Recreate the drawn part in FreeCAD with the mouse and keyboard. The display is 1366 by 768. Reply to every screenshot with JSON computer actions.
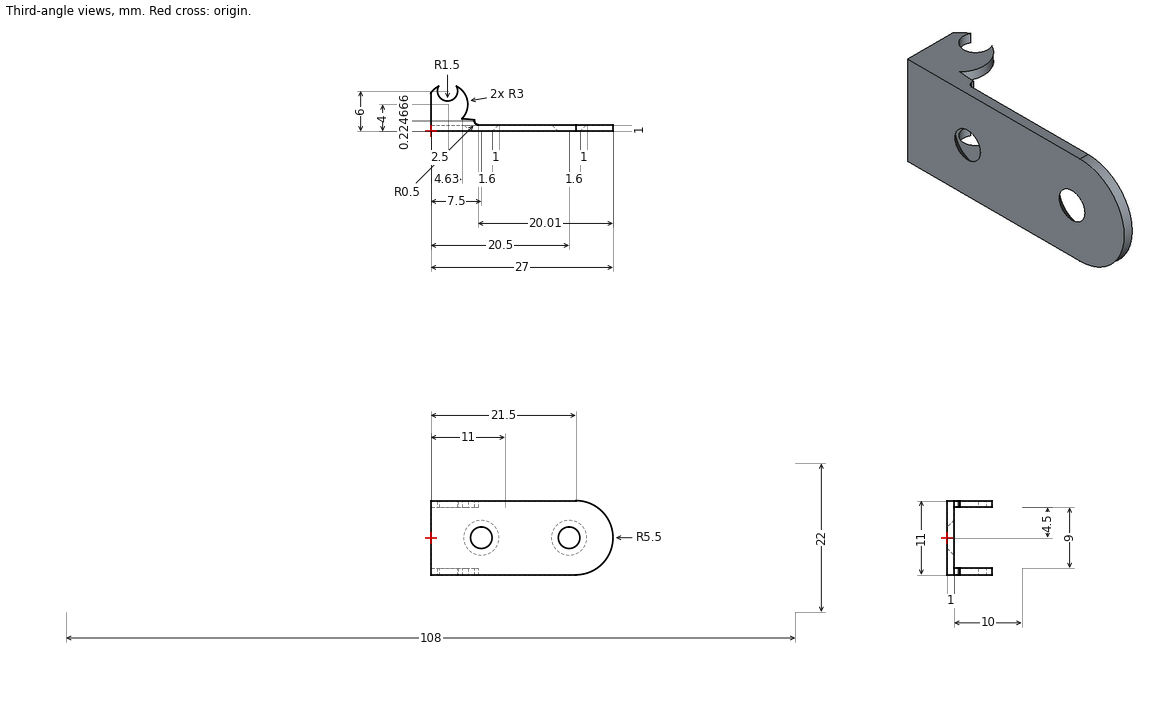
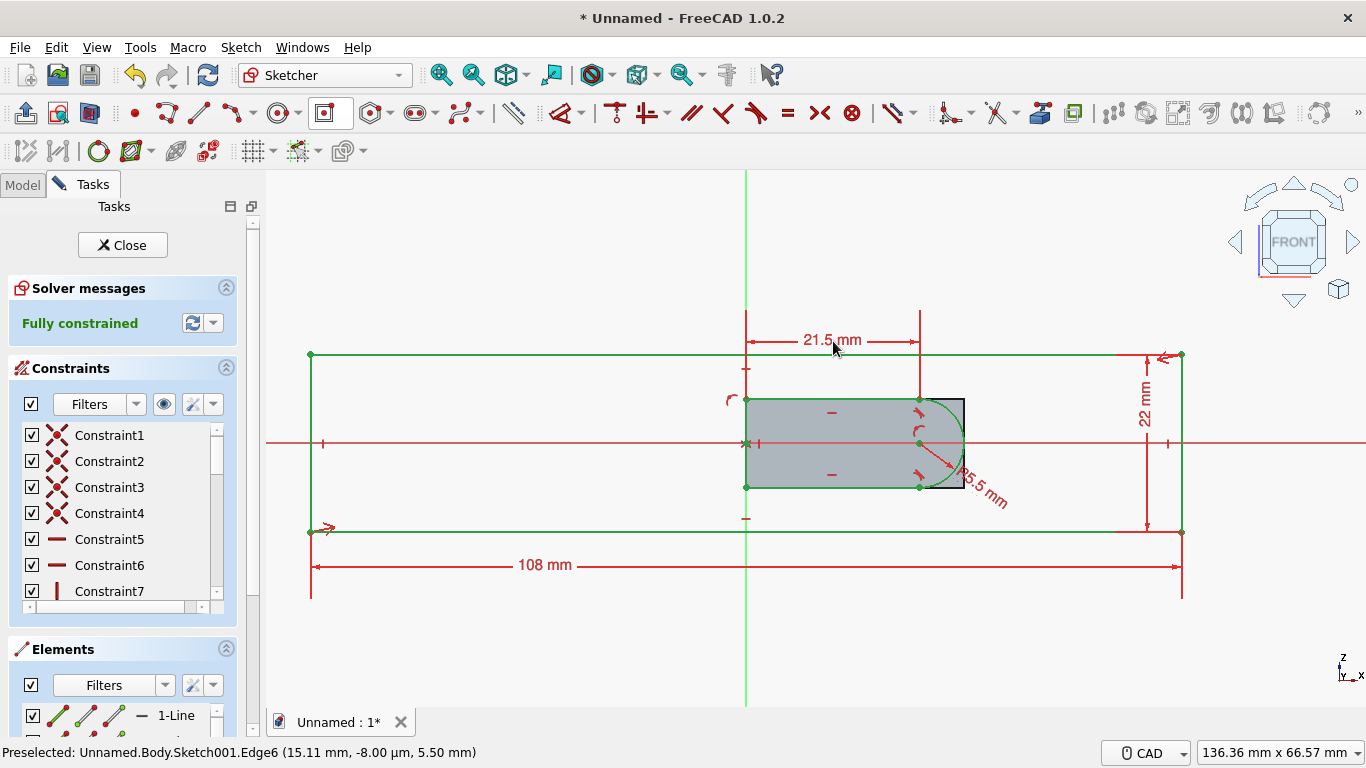
{"action": "left_click", "coordinate": [123, 245]}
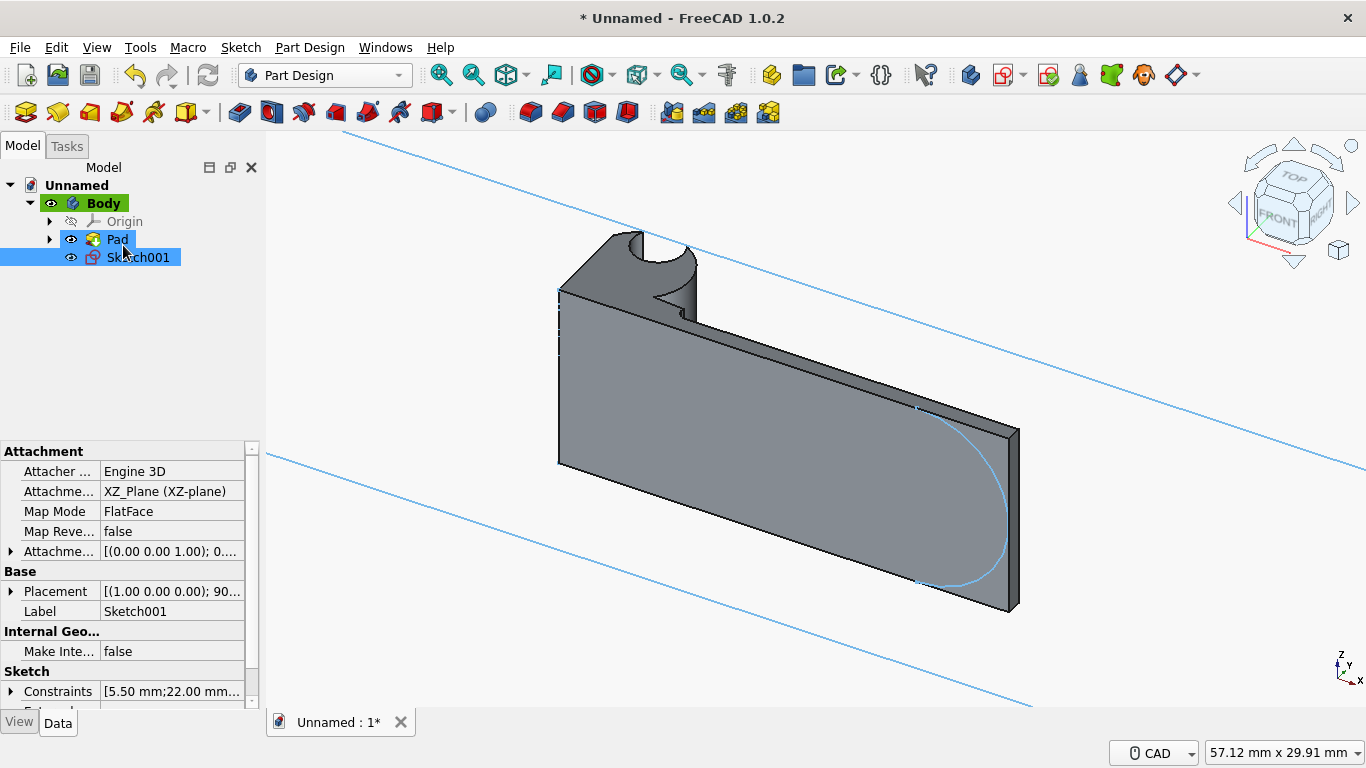
{"action": "left_click", "coordinate": [240, 112]}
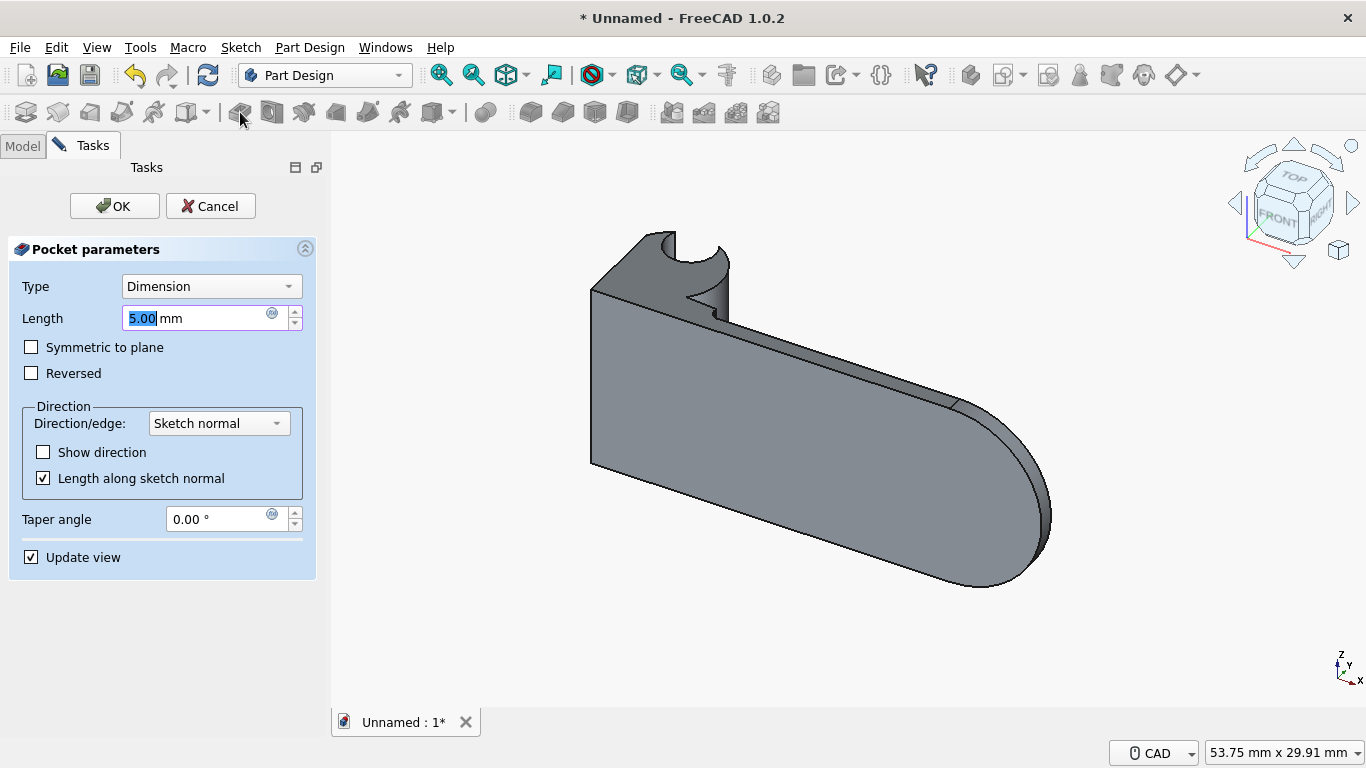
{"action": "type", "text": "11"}
{"action": "key", "text": "Tab"}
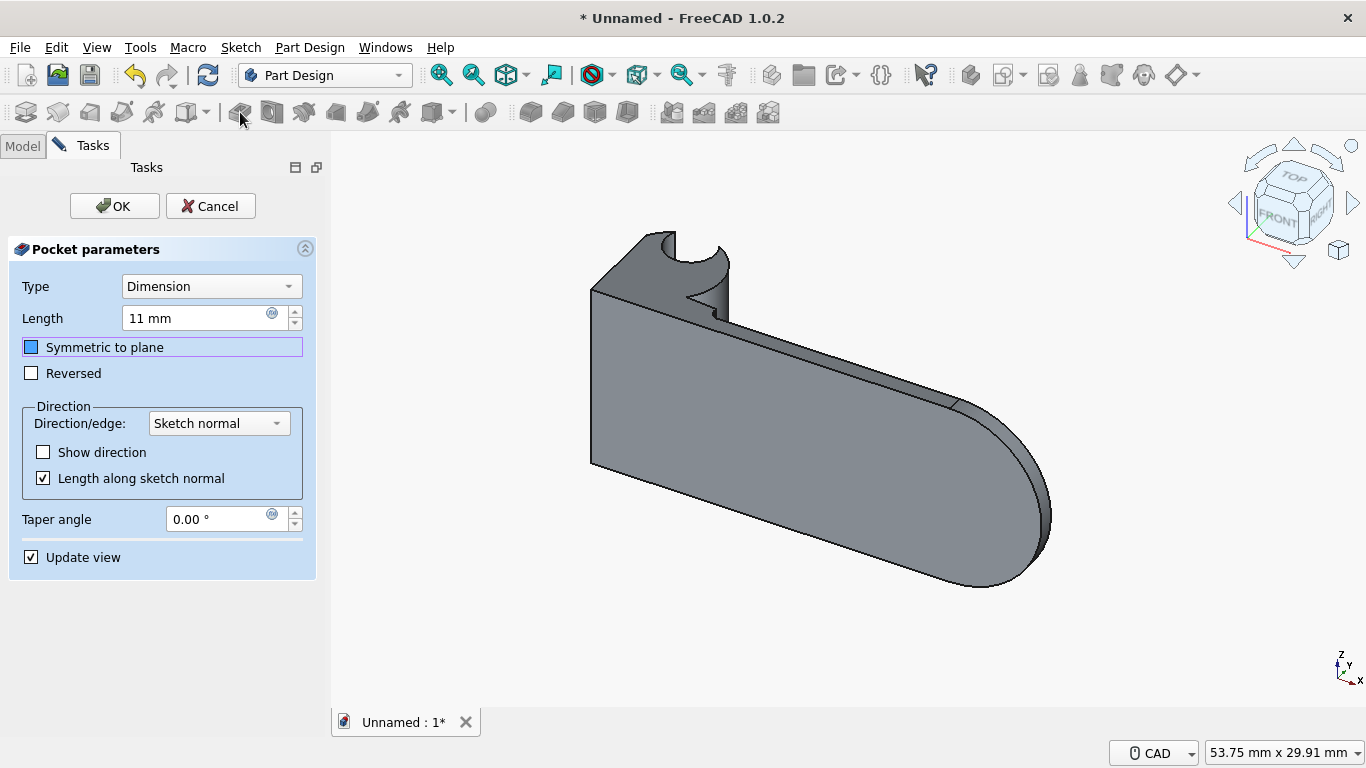
{"action": "left_click", "coordinate": [115, 206]}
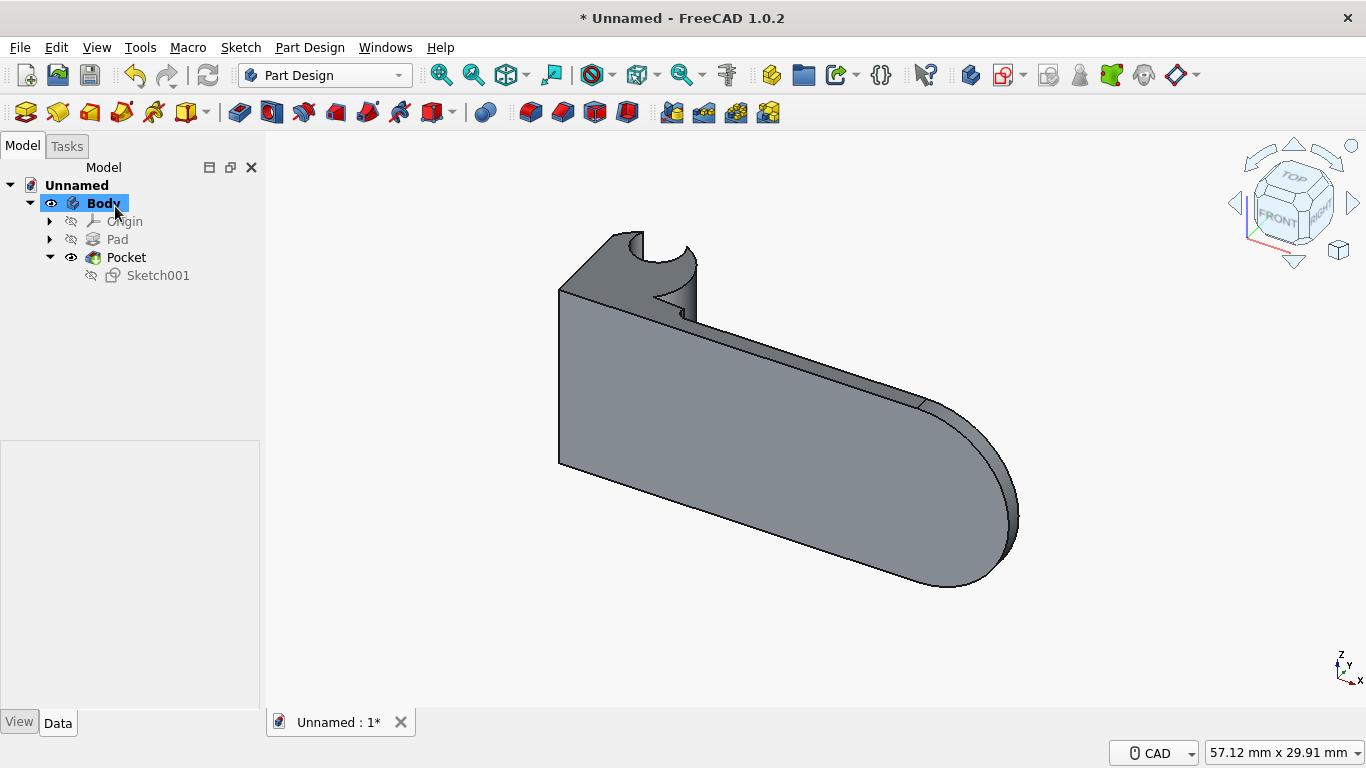
{"action": "key", "text": "6"}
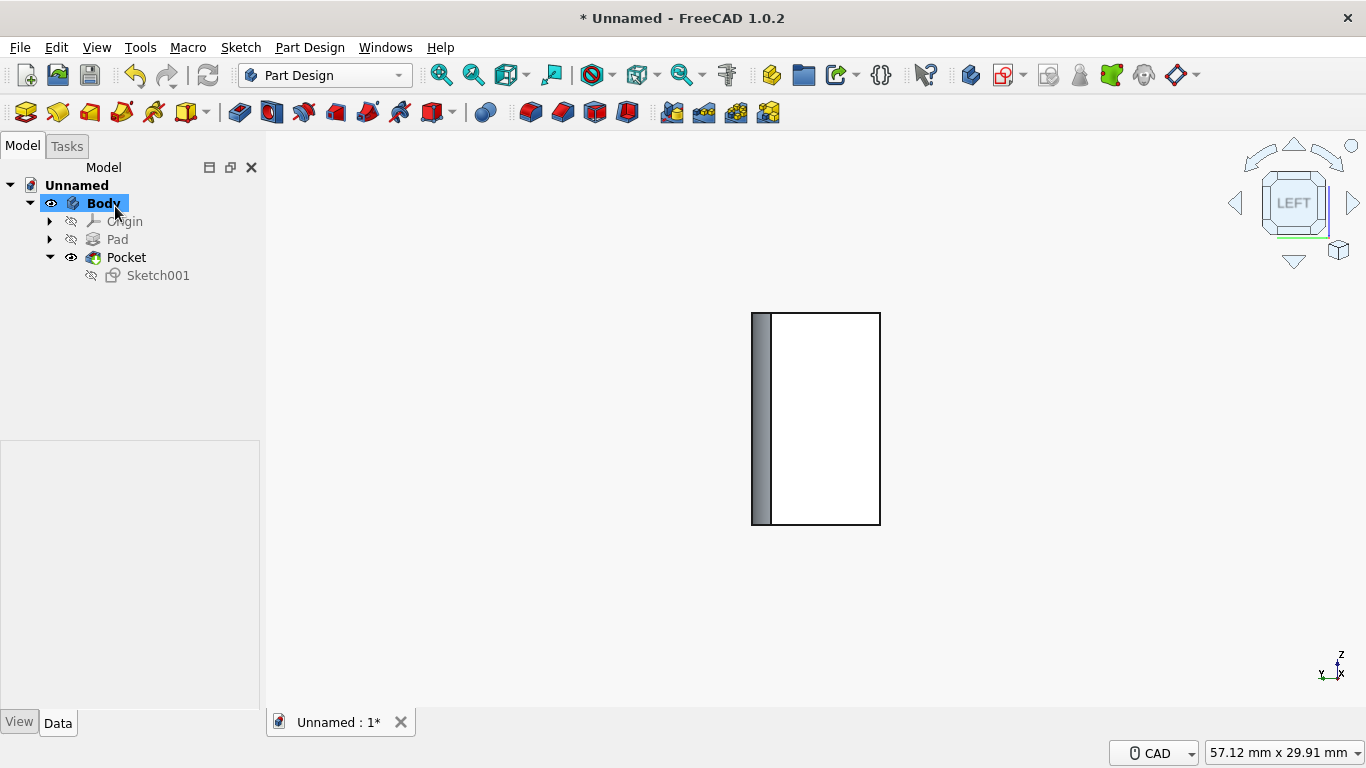
{"action": "key", "text": "v f"}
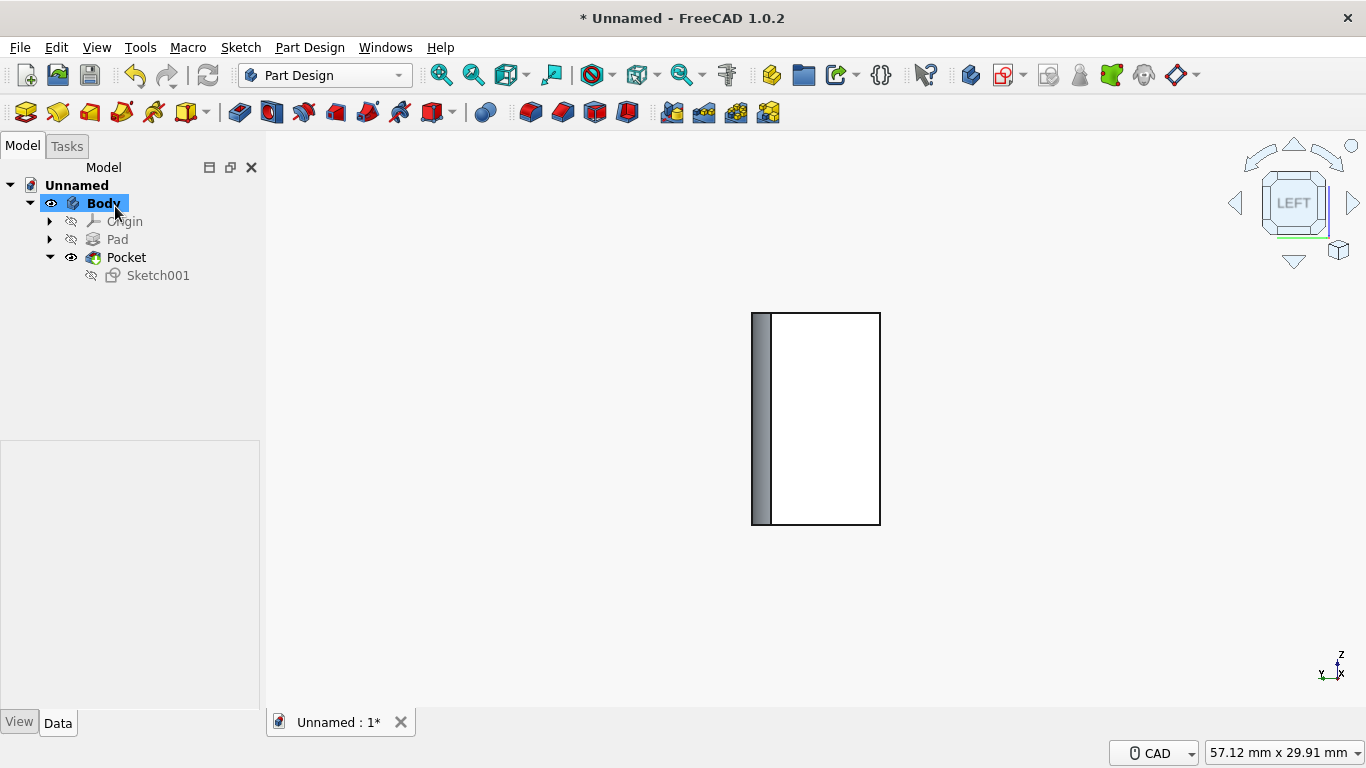
{"action": "left_click", "coordinate": [826, 388]}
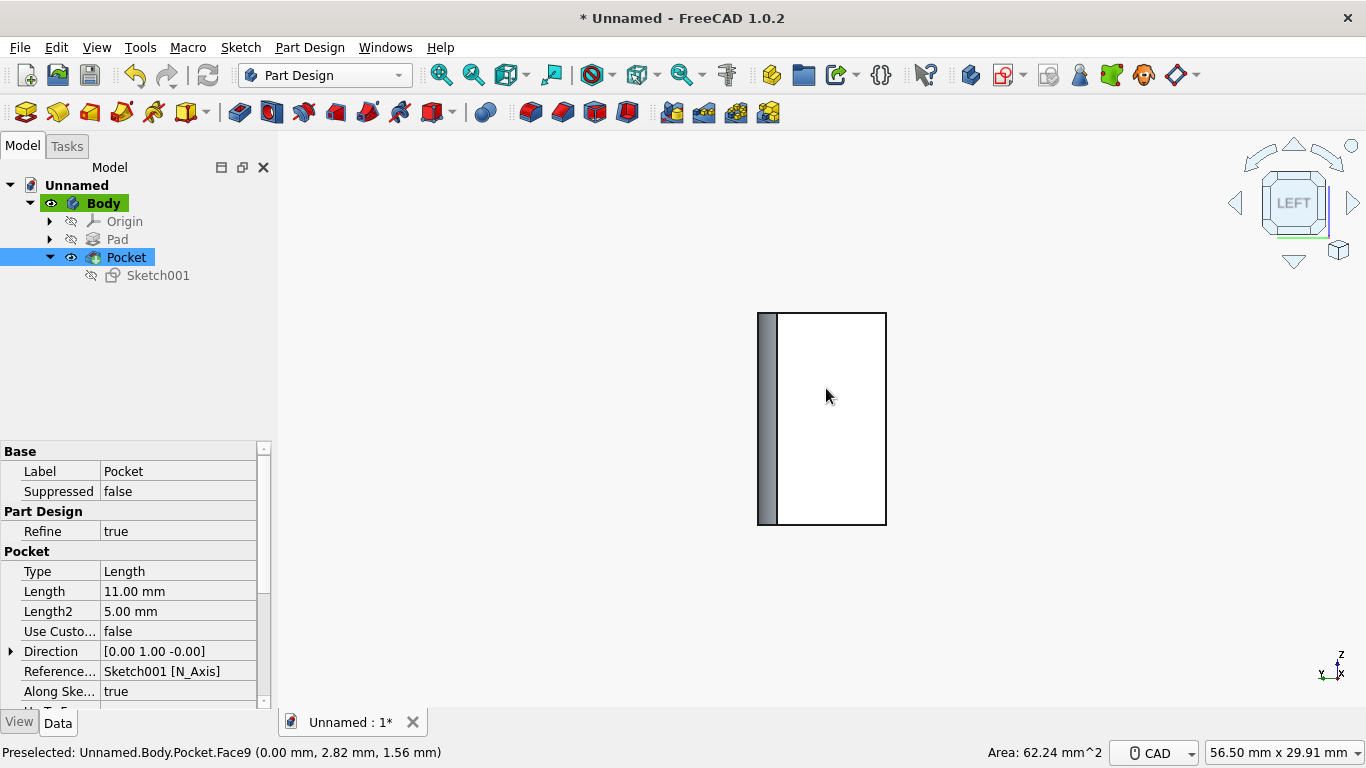
{"action": "left_click", "coordinate": [1004, 76]}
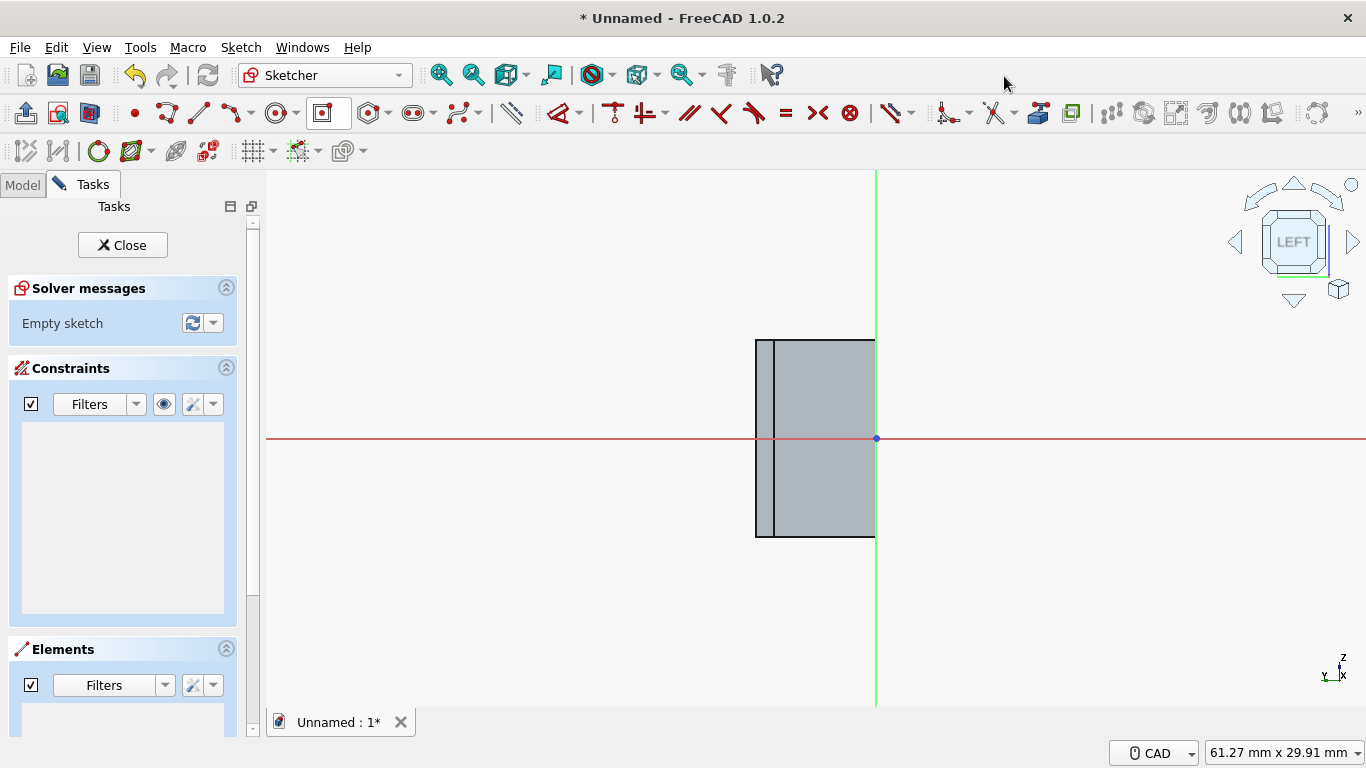
{"action": "scroll", "coordinate": [802, 438], "scroll_direction": "up", "scroll_amount": 4}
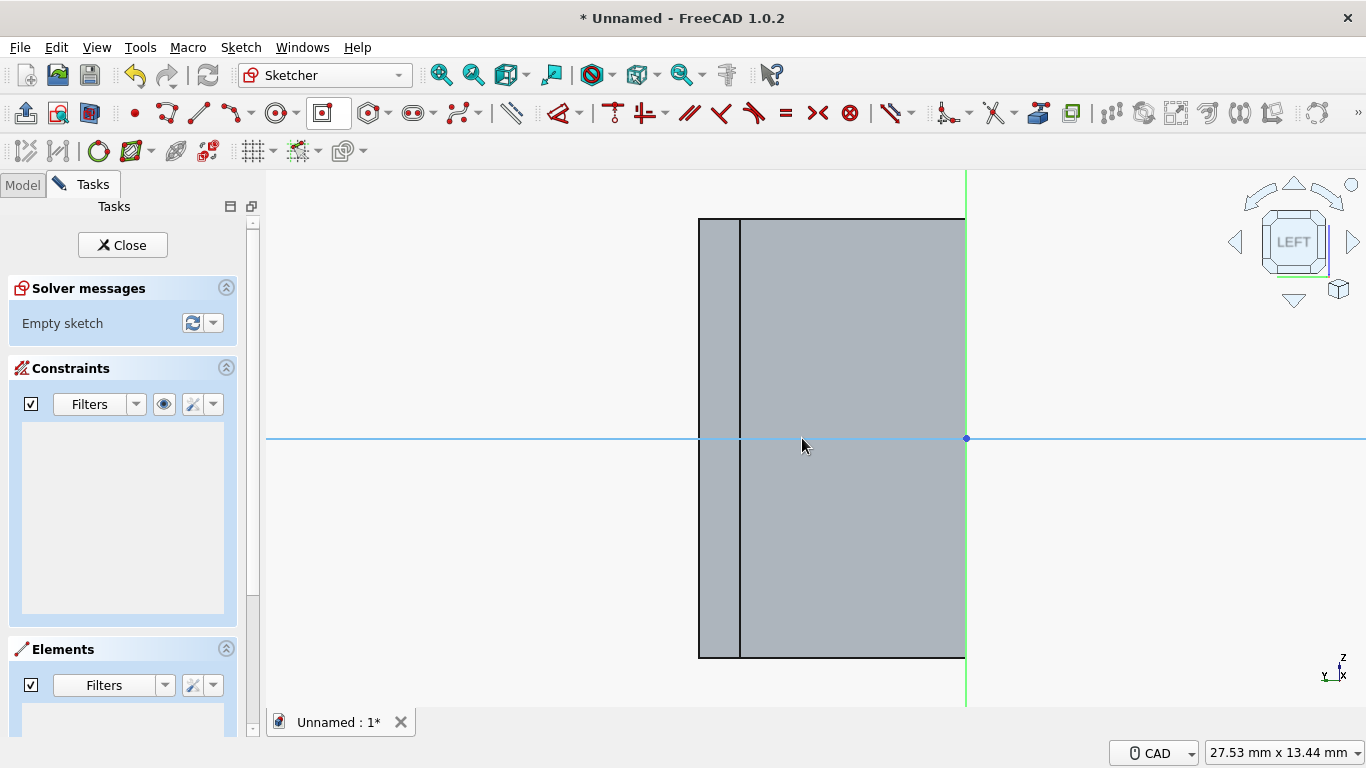
{"action": "left_click", "coordinate": [346, 114]}